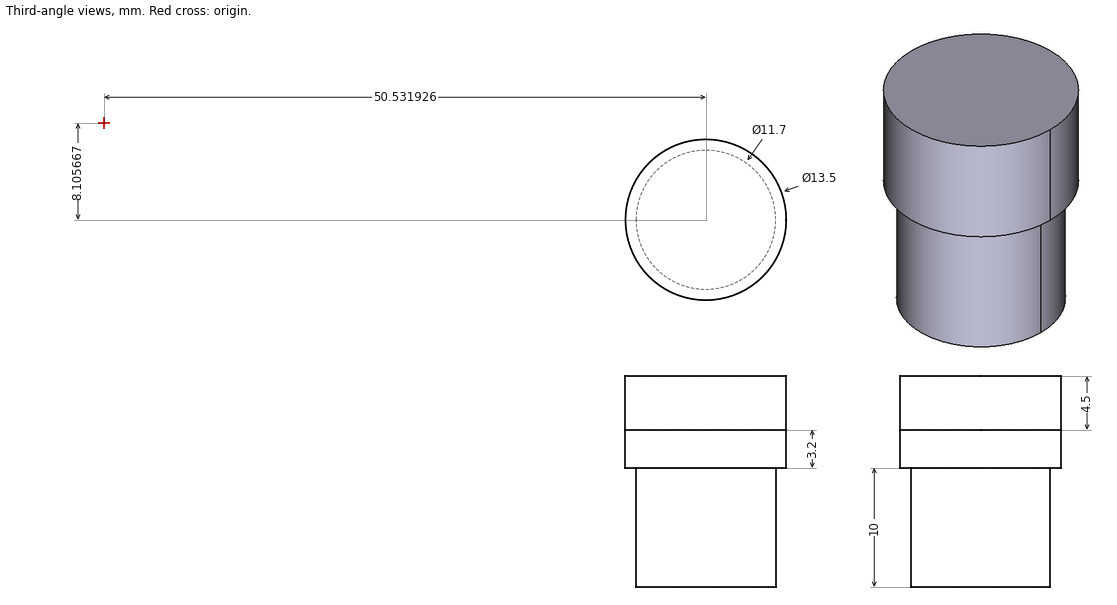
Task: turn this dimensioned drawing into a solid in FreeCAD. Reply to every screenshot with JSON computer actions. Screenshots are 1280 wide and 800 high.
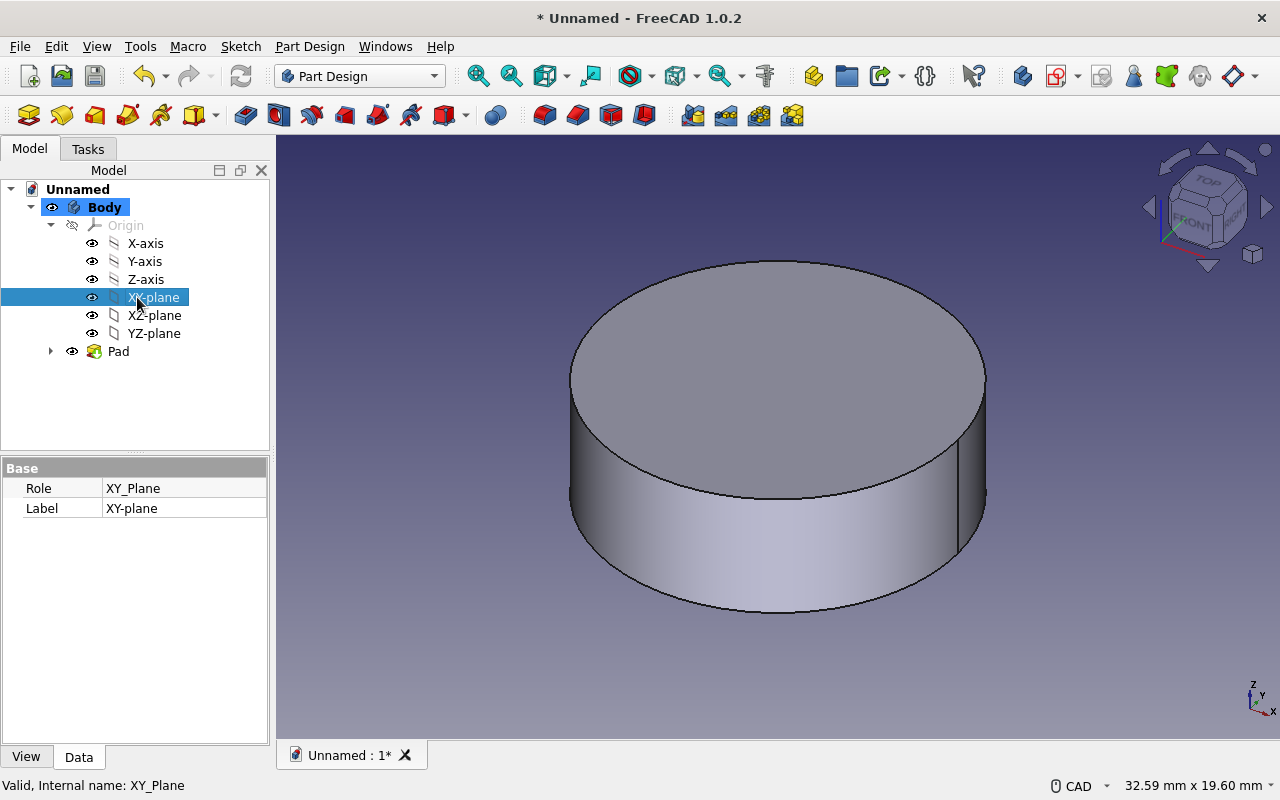
{"action": "left_click", "coordinate": [1232, 76]}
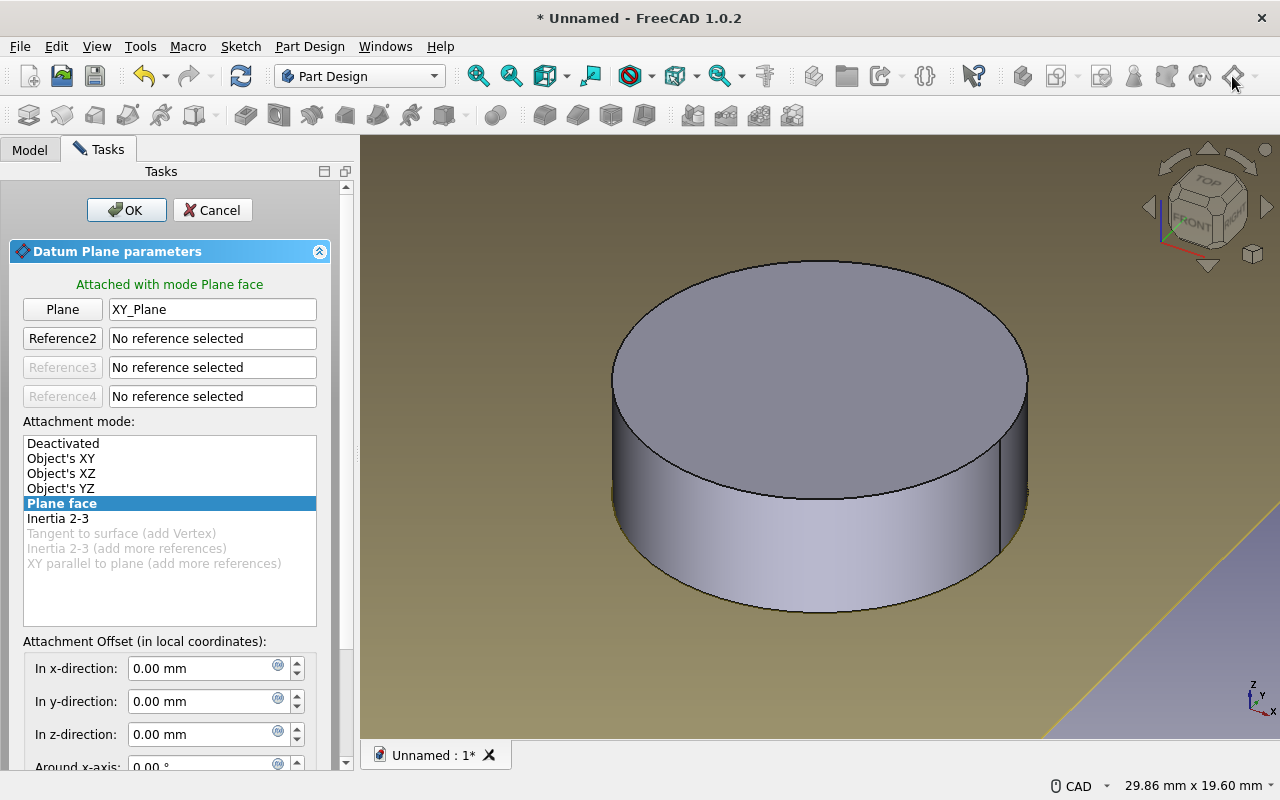
{"action": "triple_click", "coordinate": [210, 734]}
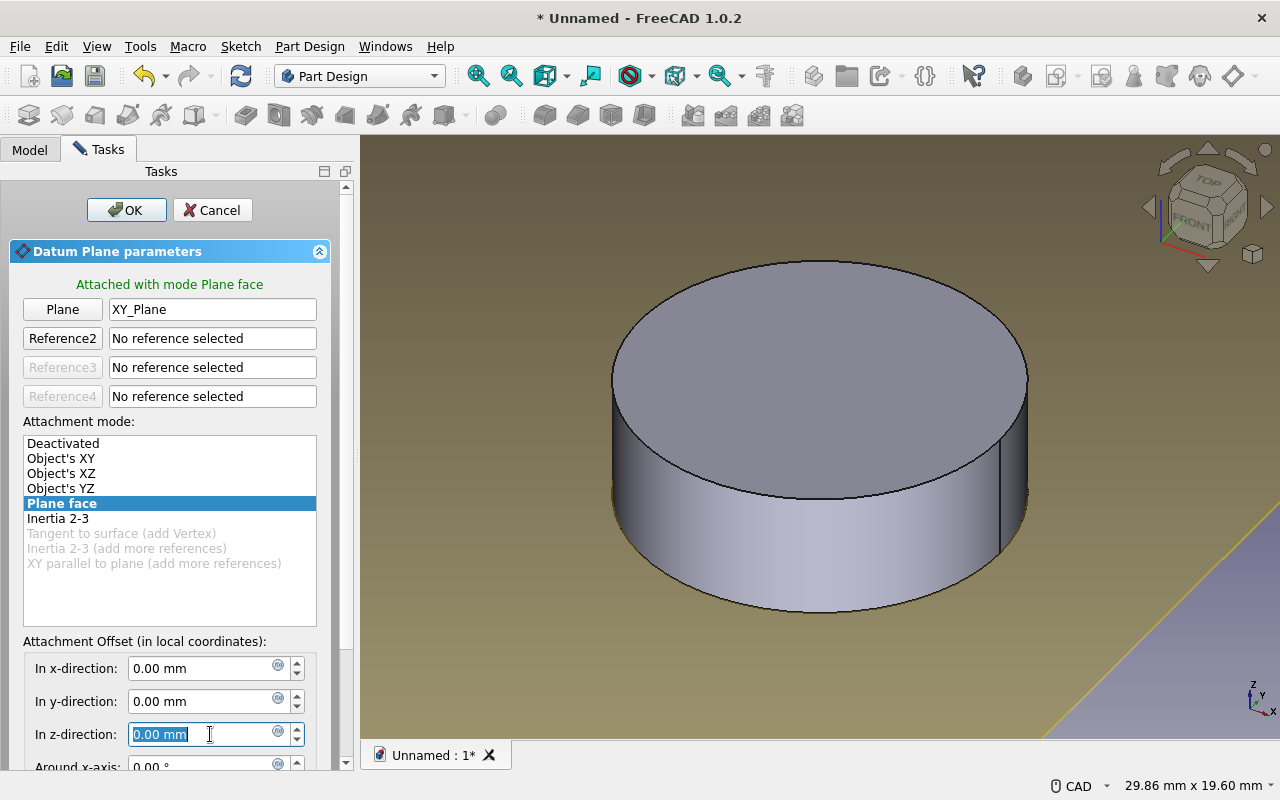
{"action": "type", "text": "-3.2"}
{"action": "key", "text": "Tab"}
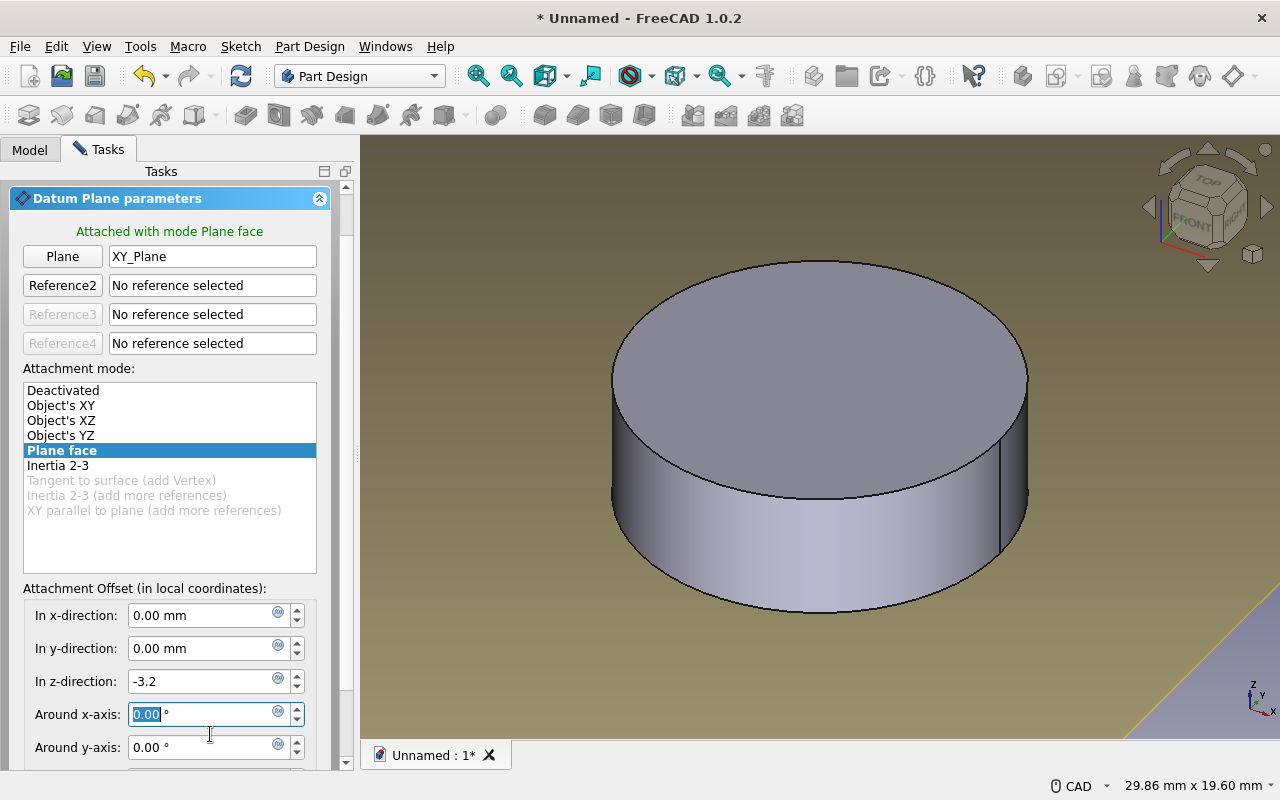
{"action": "scroll", "coordinate": [346, 476], "scroll_direction": "up", "scroll_amount": 2}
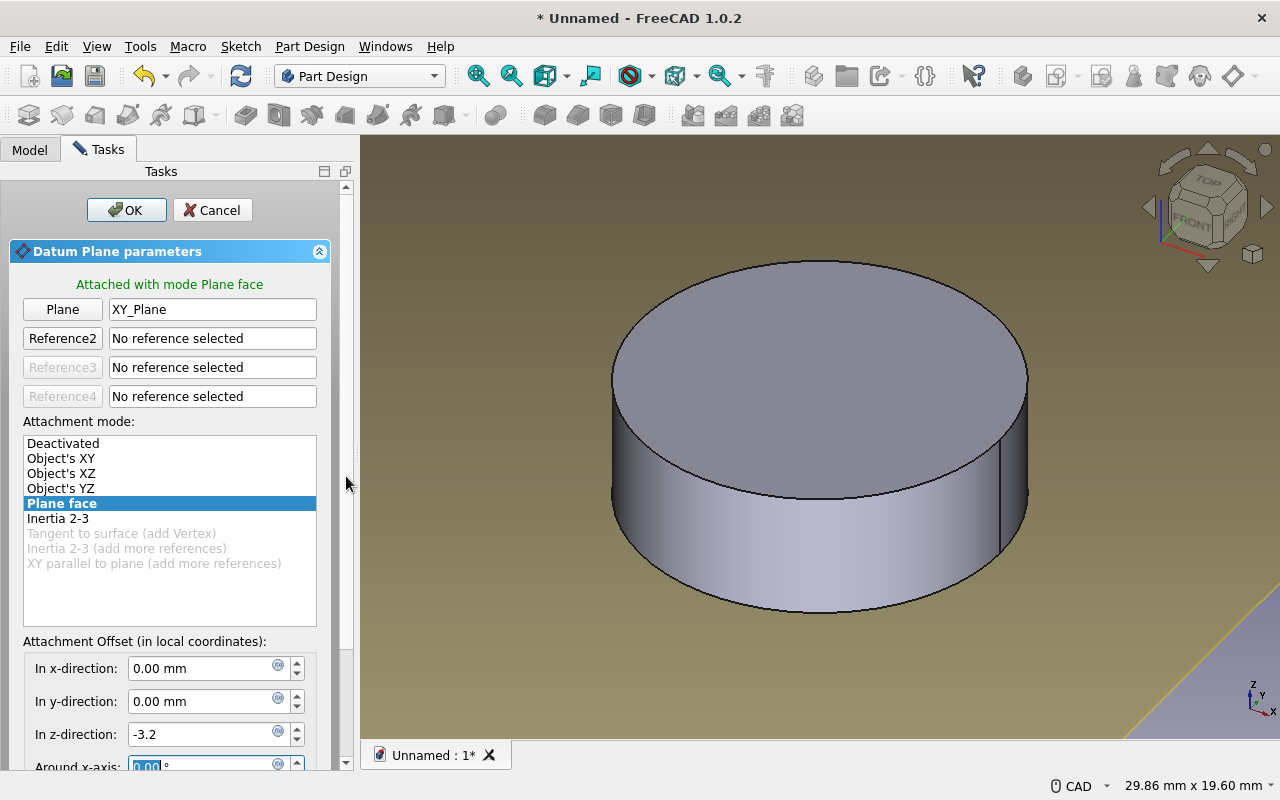
{"action": "left_click", "coordinate": [127, 210]}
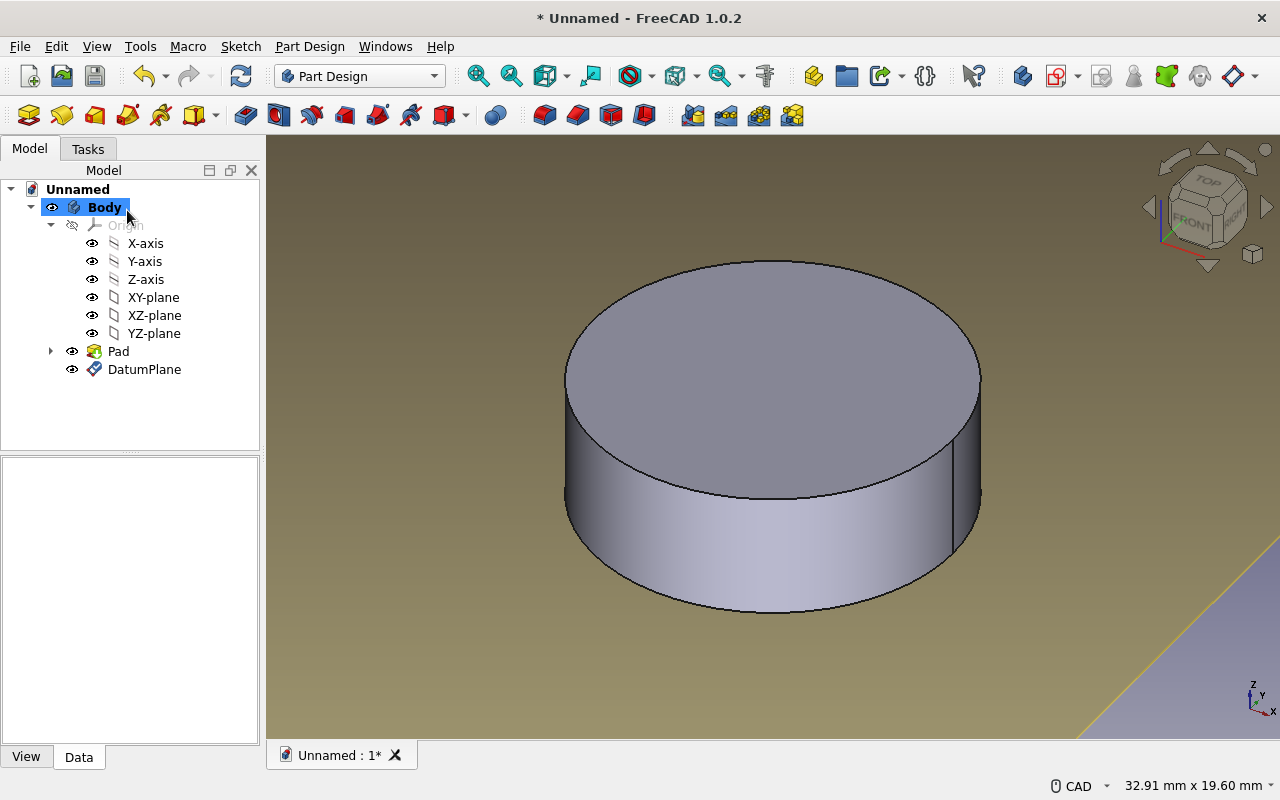
{"action": "left_click", "coordinate": [117, 369]}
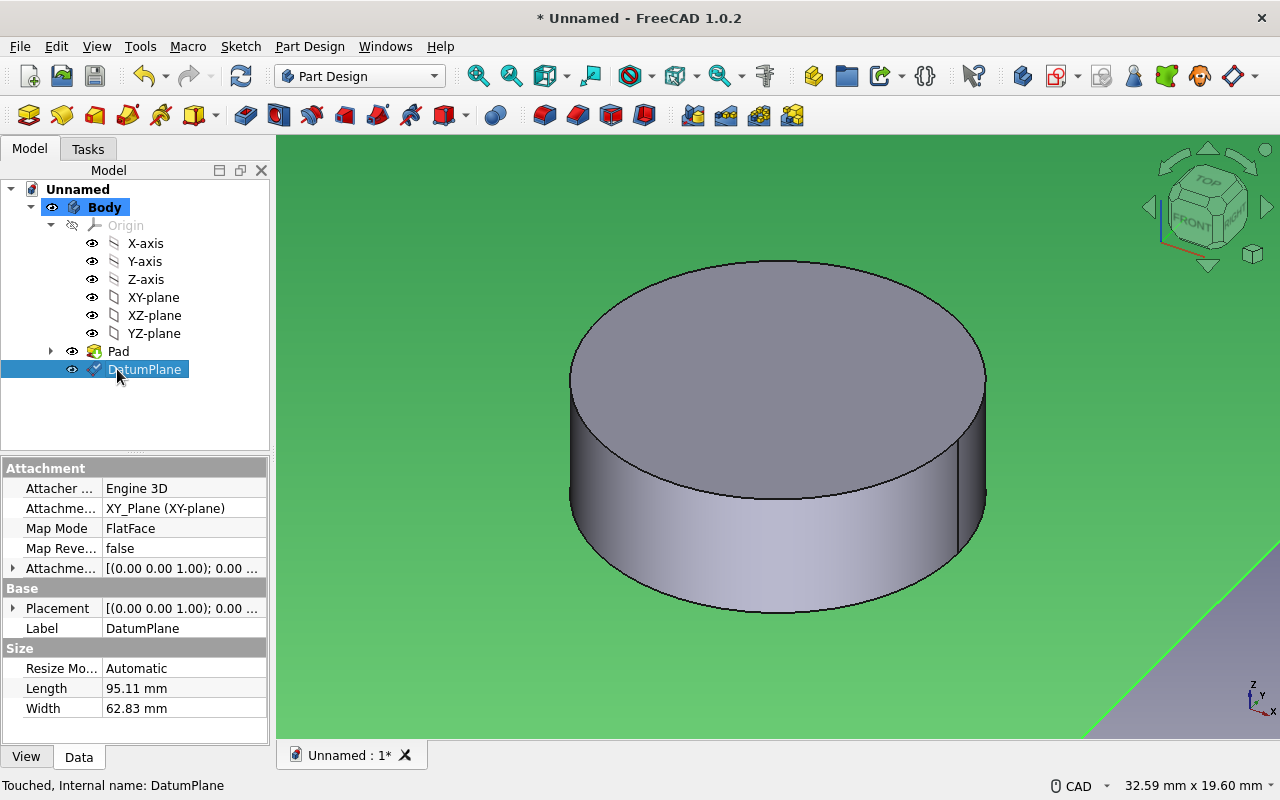
{"action": "left_click", "coordinate": [1056, 76]}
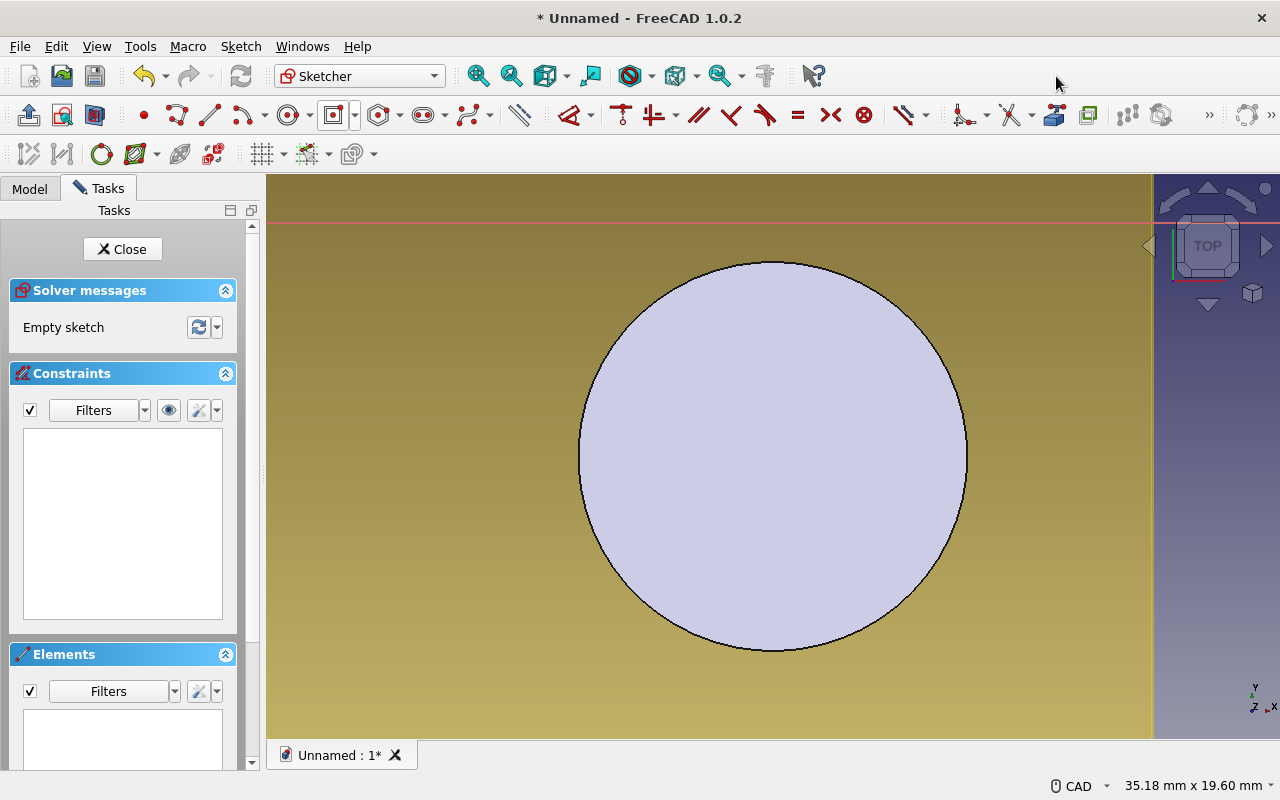
{"action": "key", "text": "q s"}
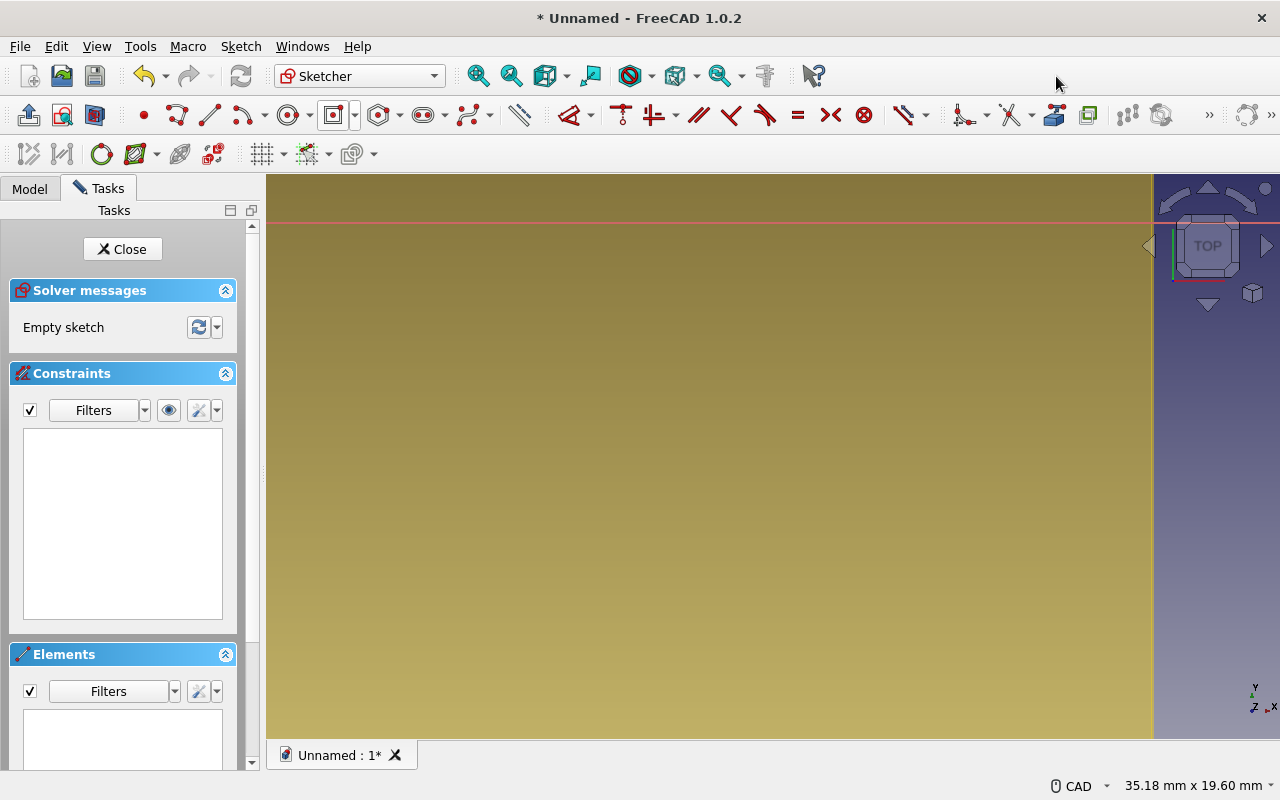
{"action": "key", "text": "g c"}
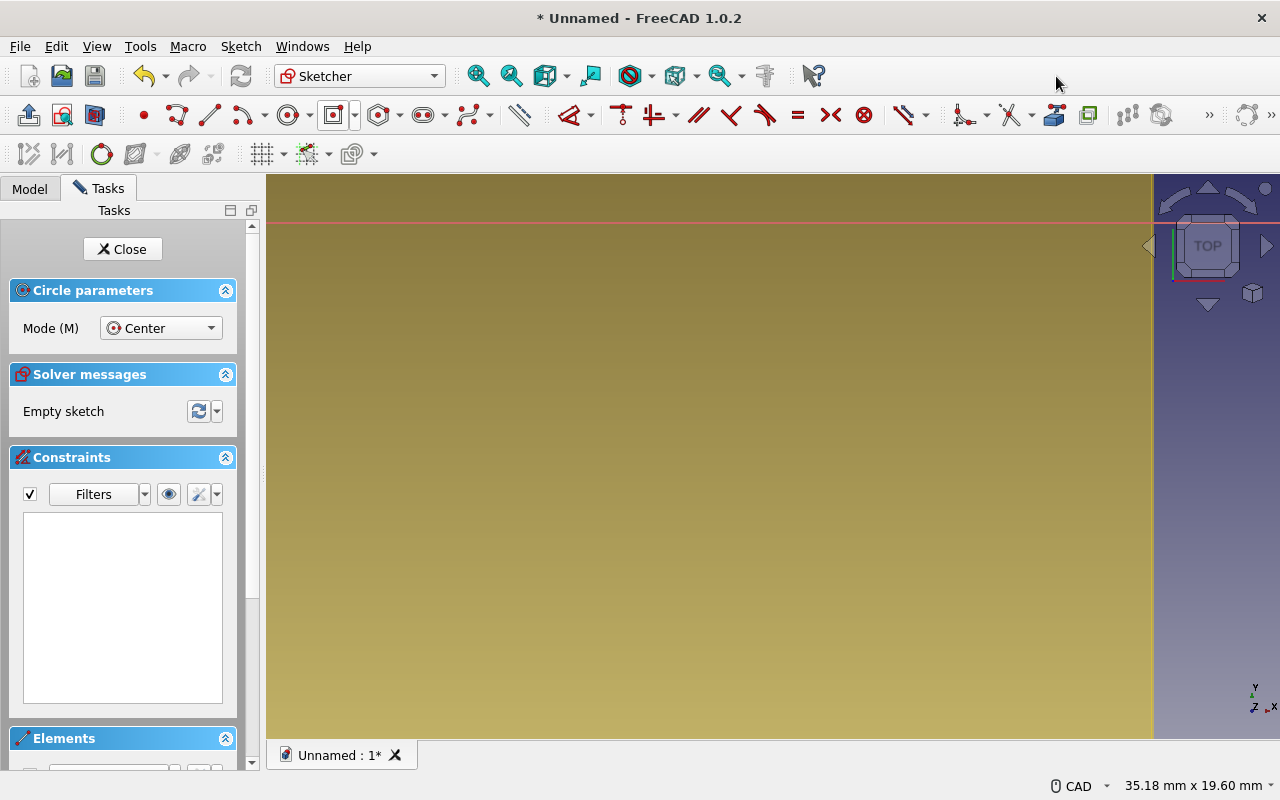
{"action": "left_click", "coordinate": [773, 456]}
{"action": "mouse_move", "coordinate": [910, 319]}